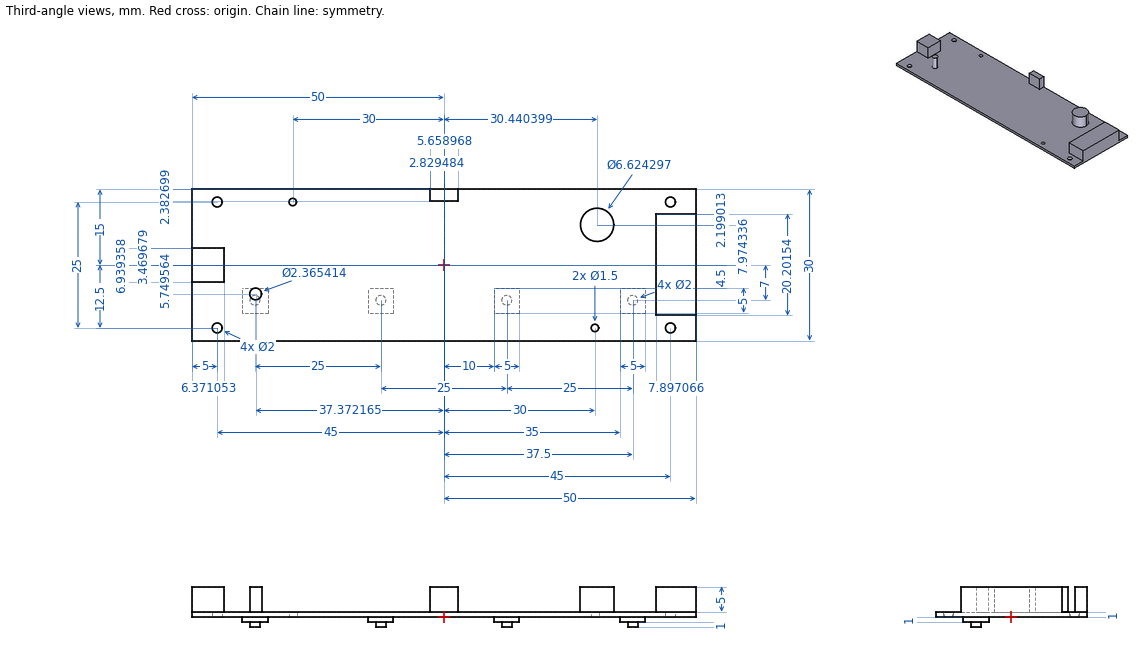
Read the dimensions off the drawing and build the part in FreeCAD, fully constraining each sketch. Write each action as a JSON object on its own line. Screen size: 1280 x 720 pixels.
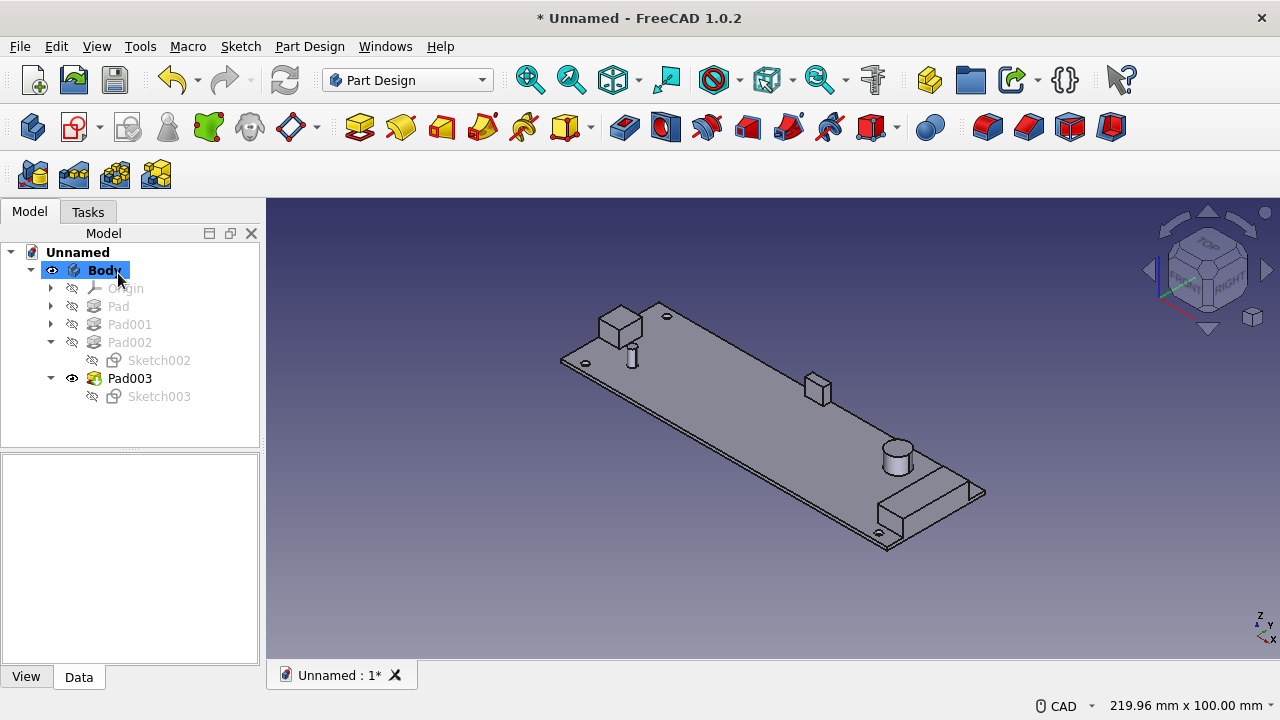
{"action": "left_click", "coordinate": [726, 397]}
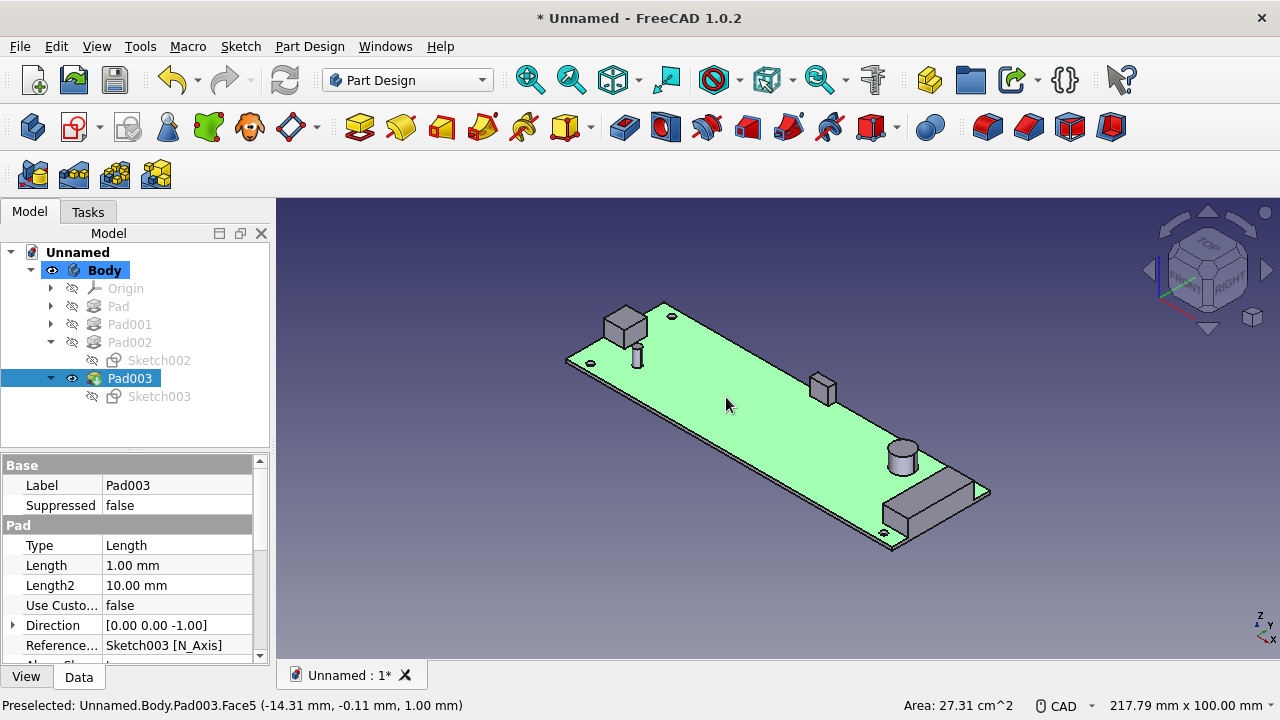
{"action": "left_click", "coordinate": [74, 128]}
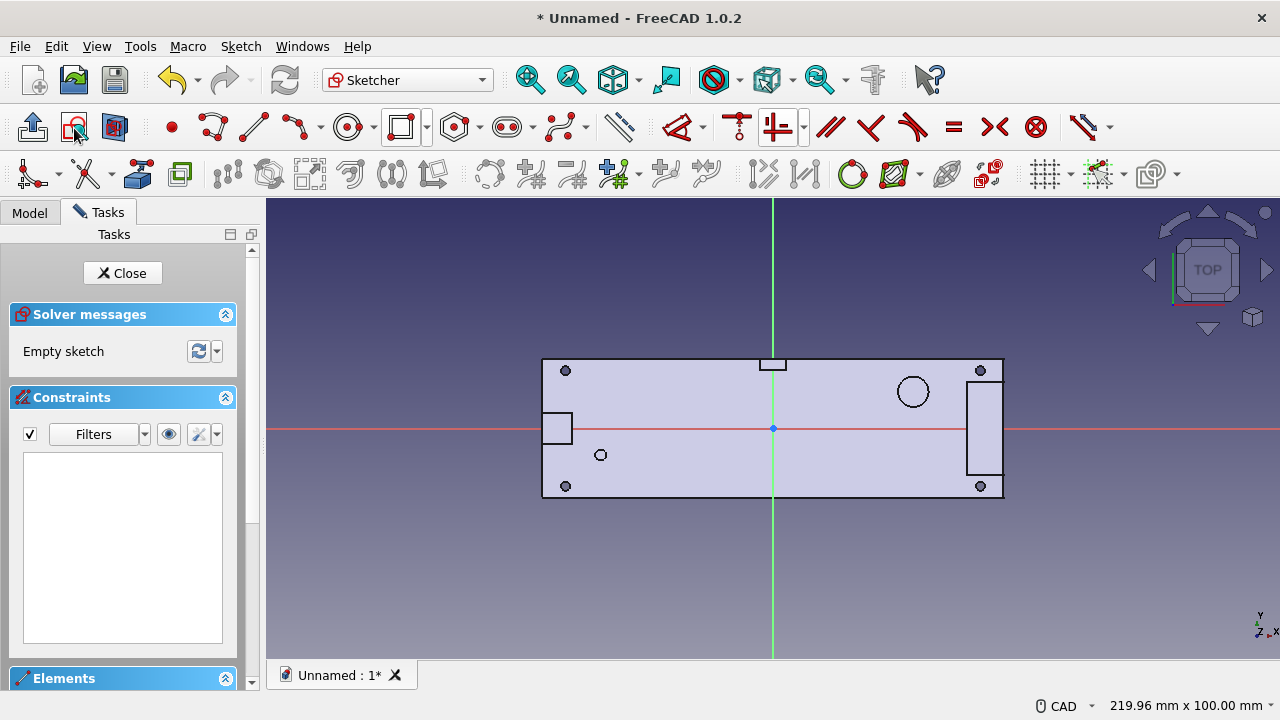
{"action": "scroll", "coordinate": [829, 428], "scroll_direction": "up", "scroll_amount": 4}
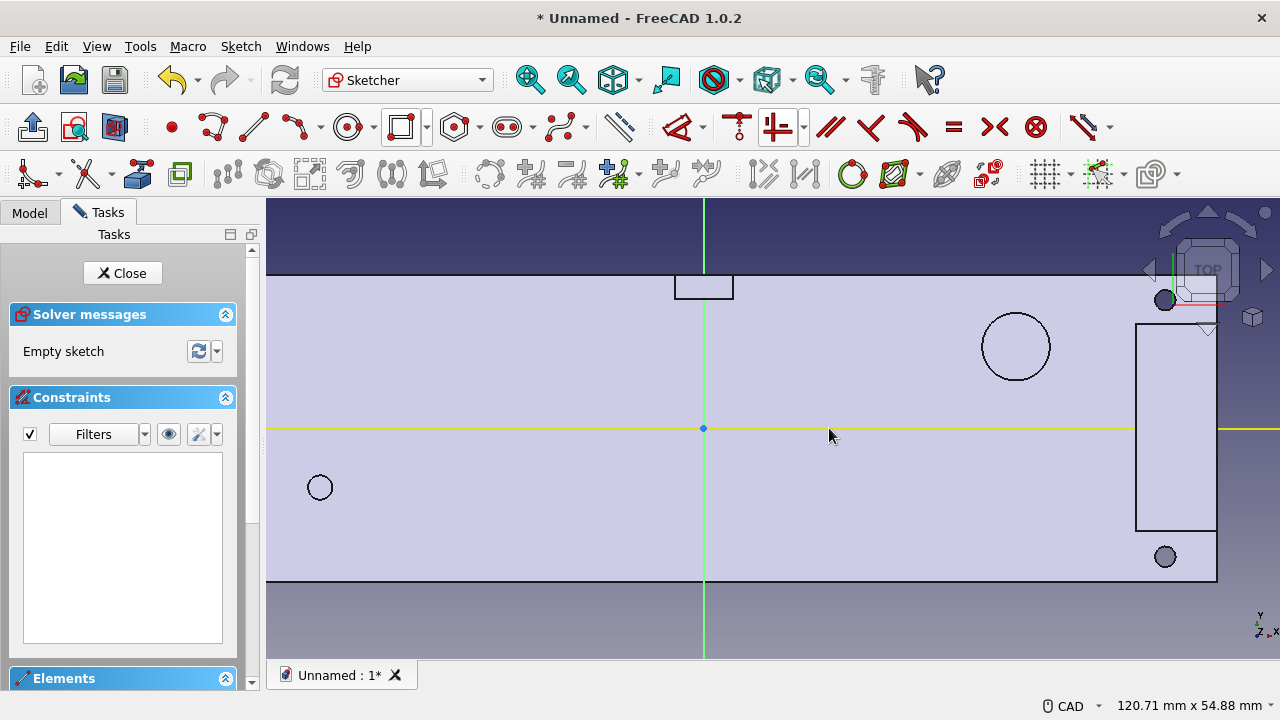
{"action": "left_click", "coordinate": [348, 128]}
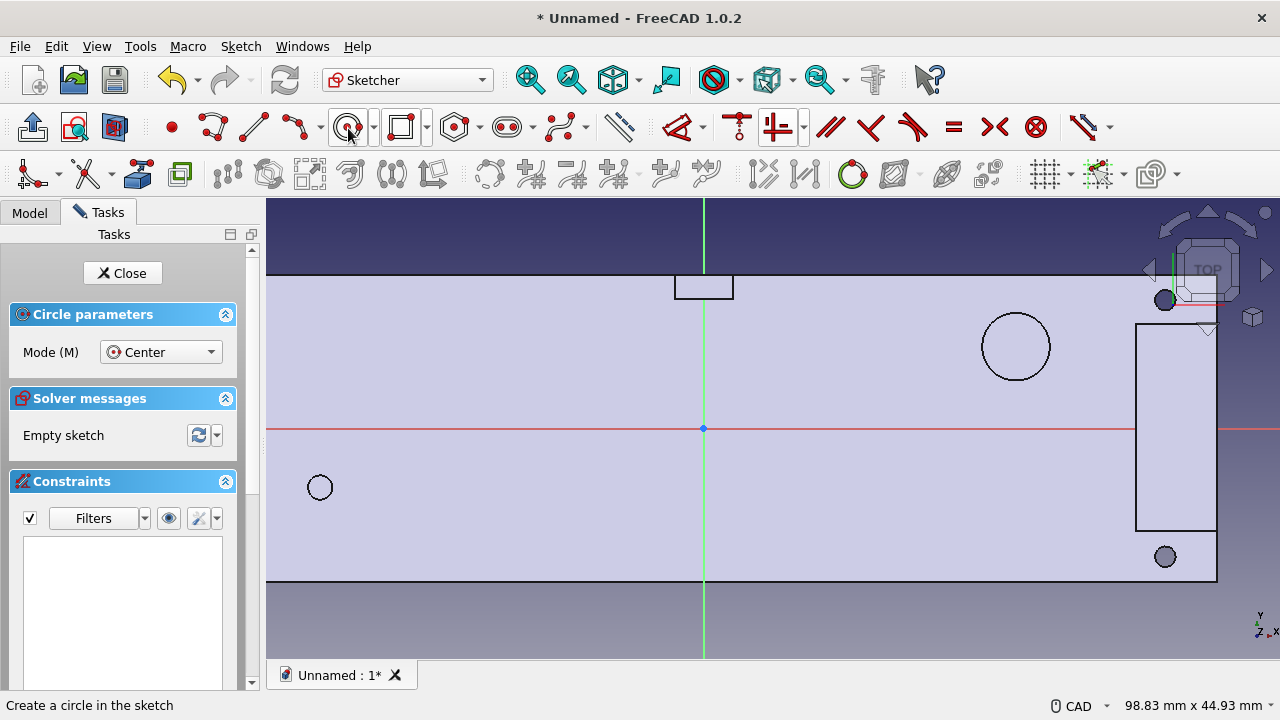
{"action": "scroll", "coordinate": [1011, 557], "scroll_direction": "up", "scroll_amount": 6}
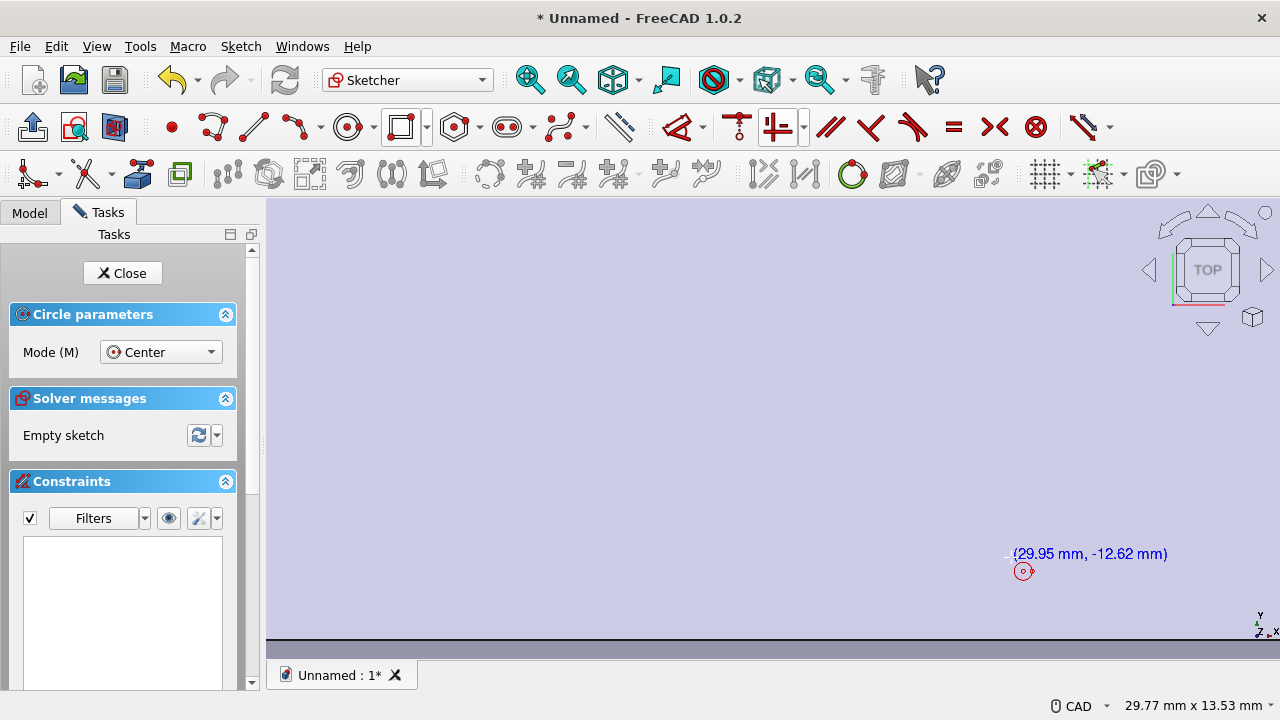
{"action": "left_click", "coordinate": [1011, 554]}
{"action": "left_click", "coordinate": [1029, 536]}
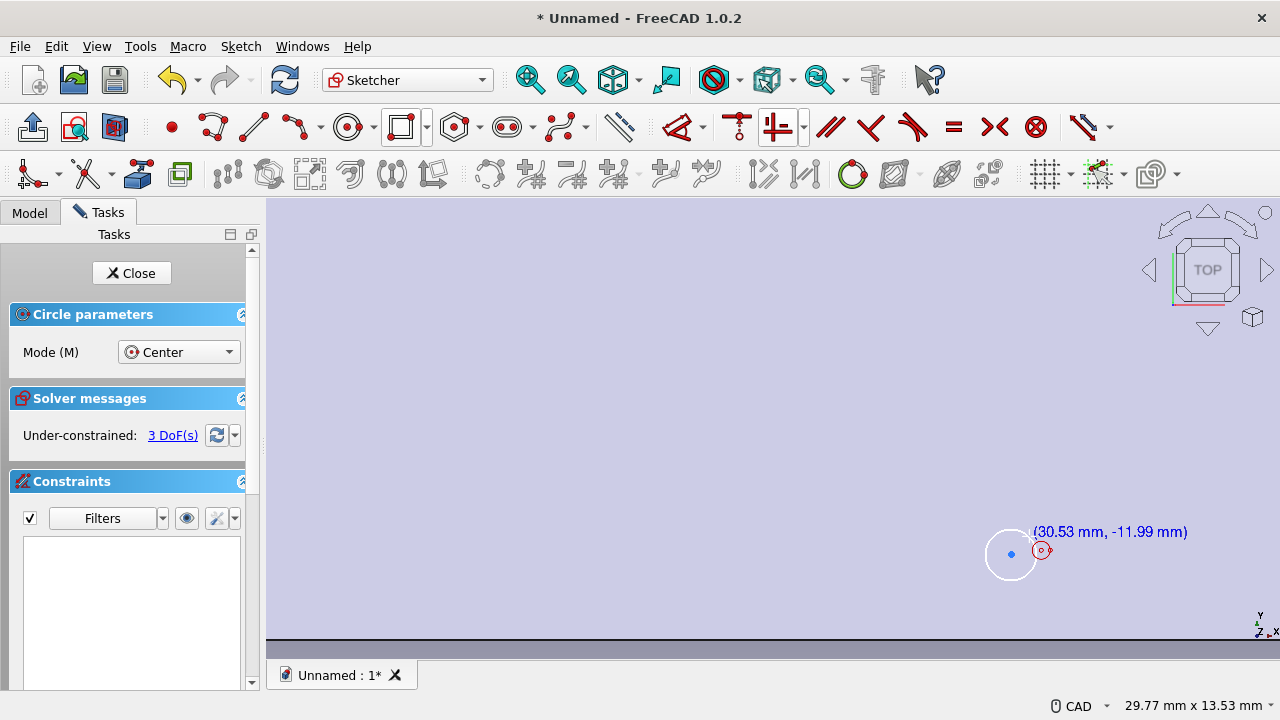
{"action": "scroll", "coordinate": [1013, 558], "scroll_direction": "down", "scroll_amount": 6}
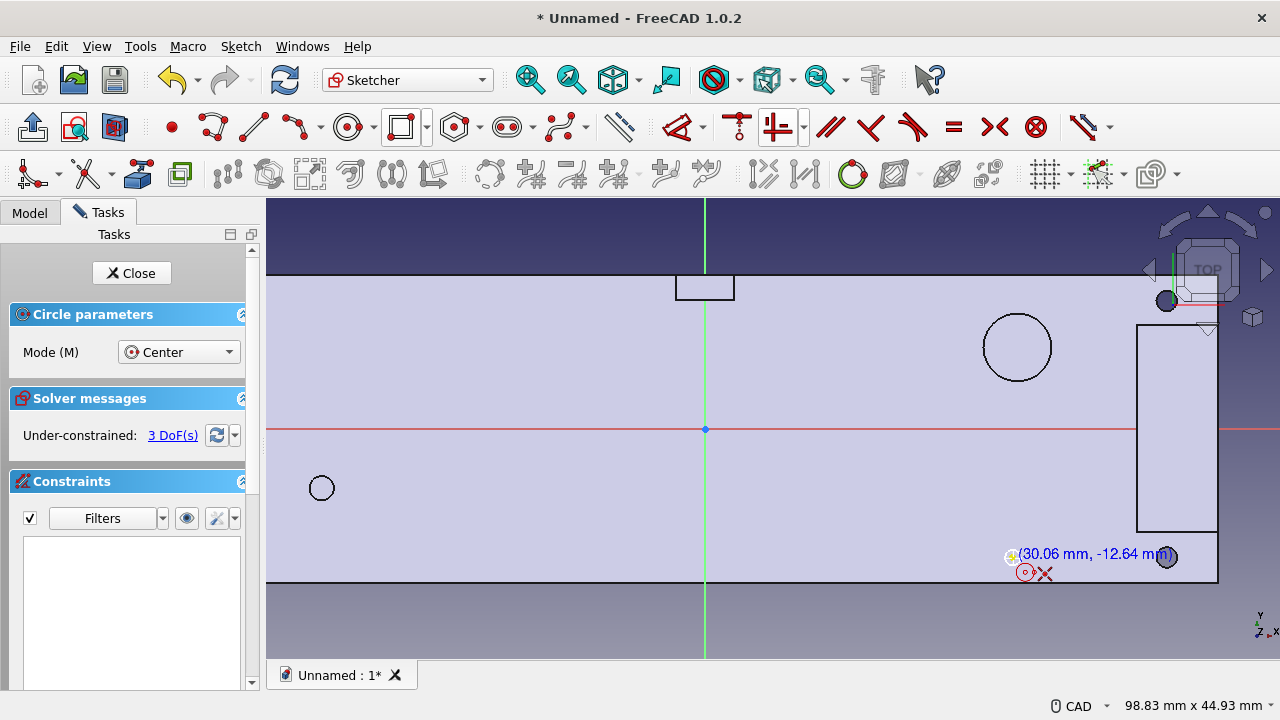
{"action": "scroll", "coordinate": [397, 301], "scroll_direction": "up", "scroll_amount": 6}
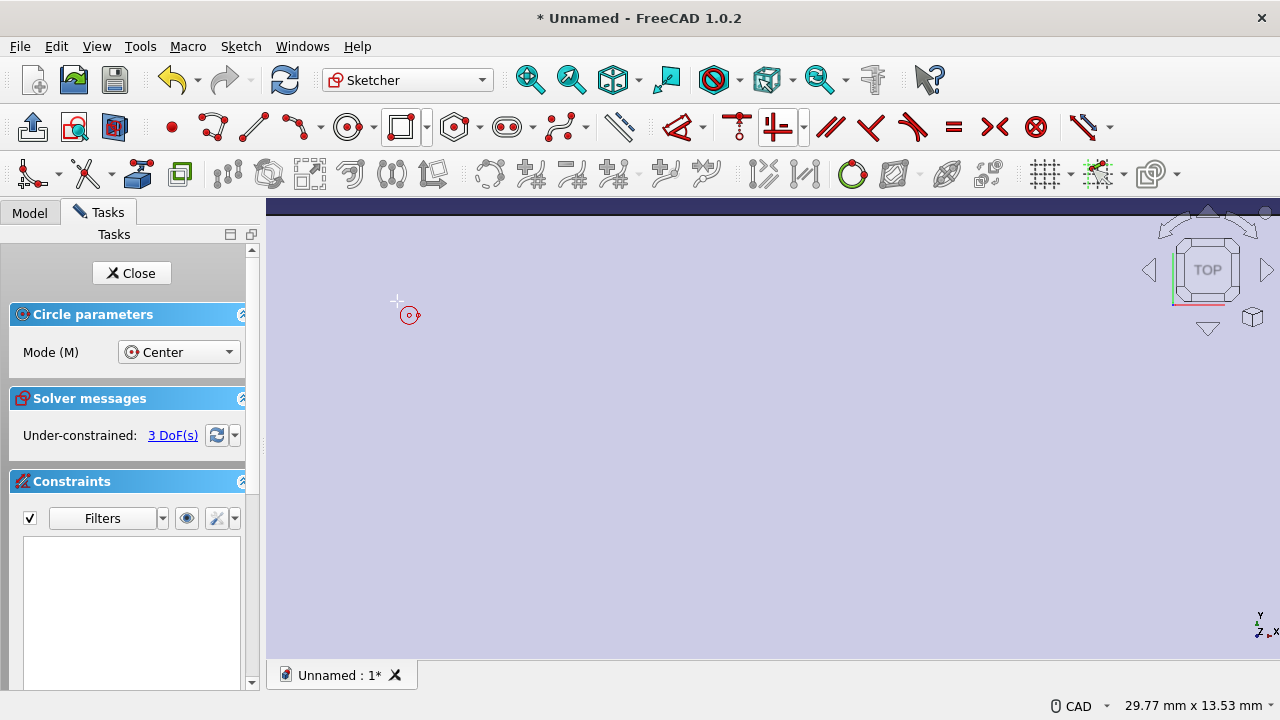
{"action": "left_click", "coordinate": [398, 300]}
{"action": "left_click", "coordinate": [416, 282]}
{"action": "key", "text": "Escape"}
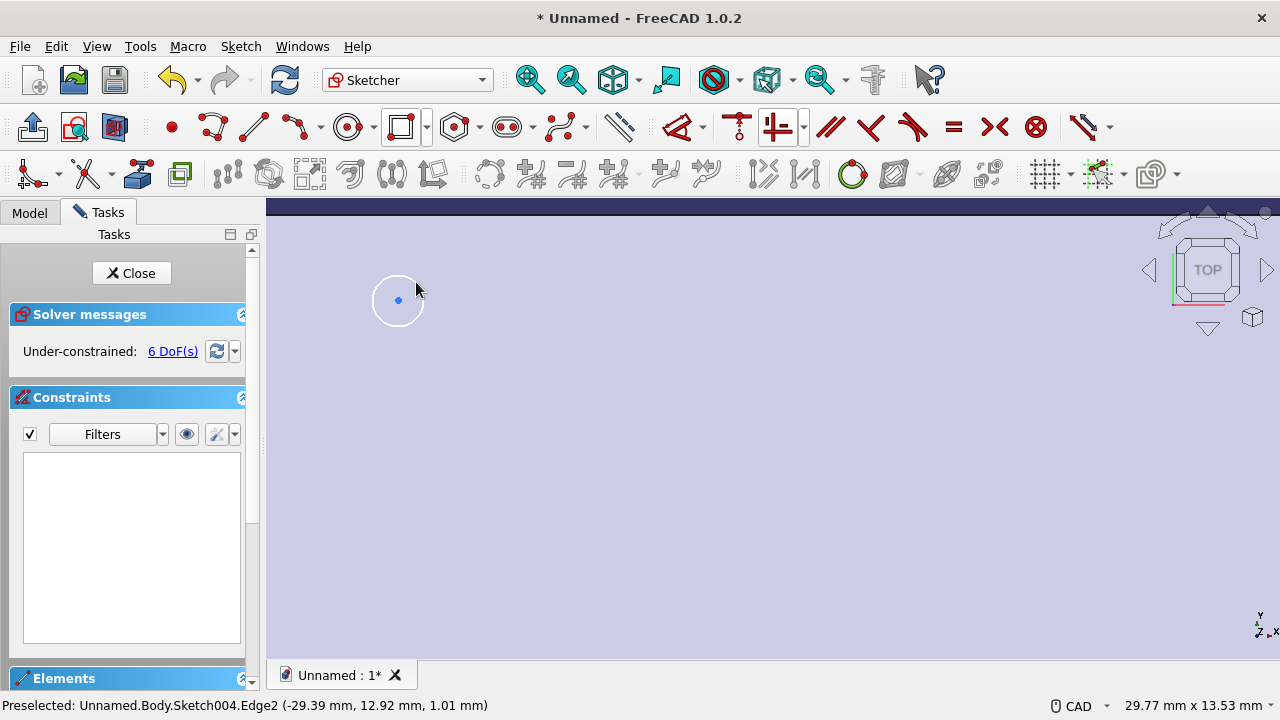
{"action": "scroll", "coordinate": [396, 300], "scroll_direction": "down", "scroll_amount": 6}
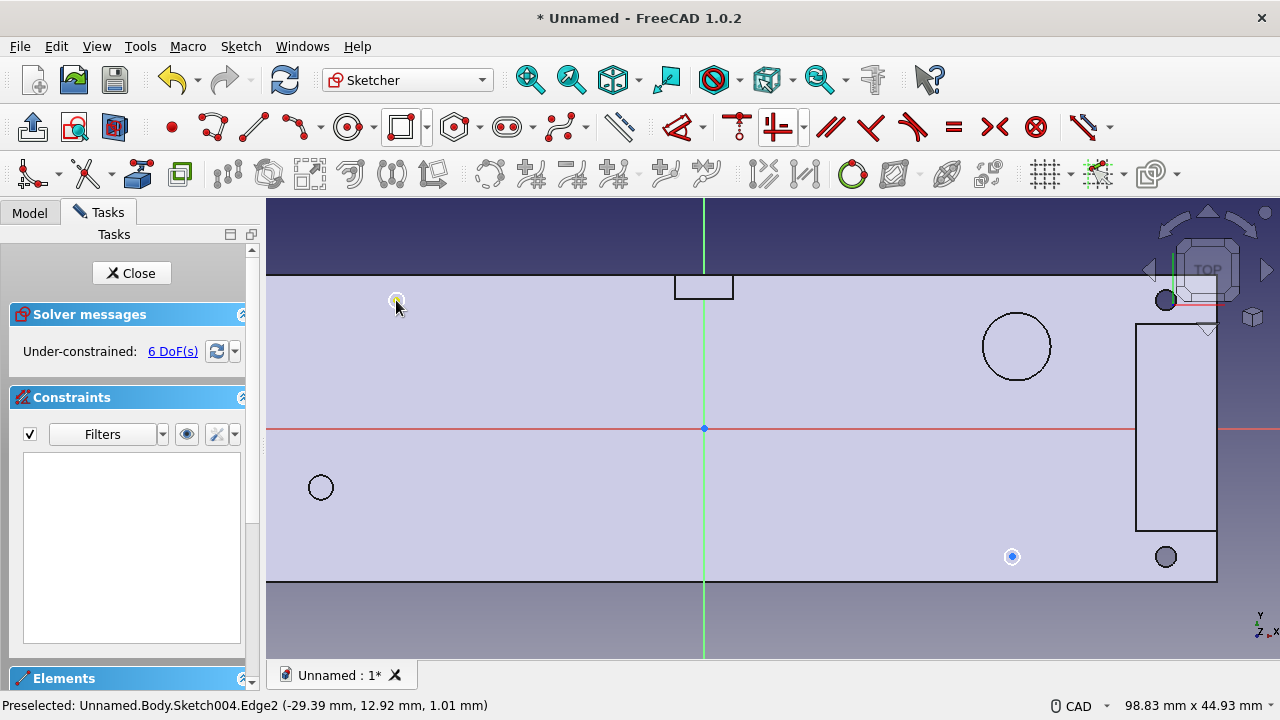
{"action": "scroll", "coordinate": [1018, 552], "scroll_direction": "up", "scroll_amount": 3}